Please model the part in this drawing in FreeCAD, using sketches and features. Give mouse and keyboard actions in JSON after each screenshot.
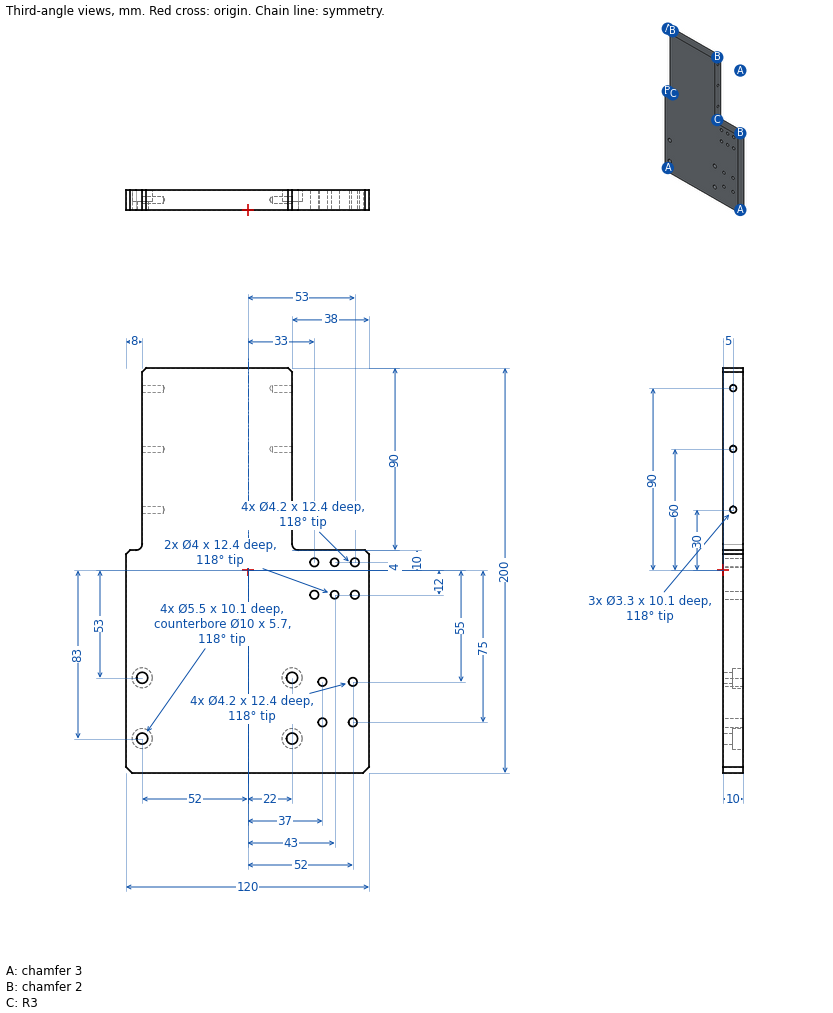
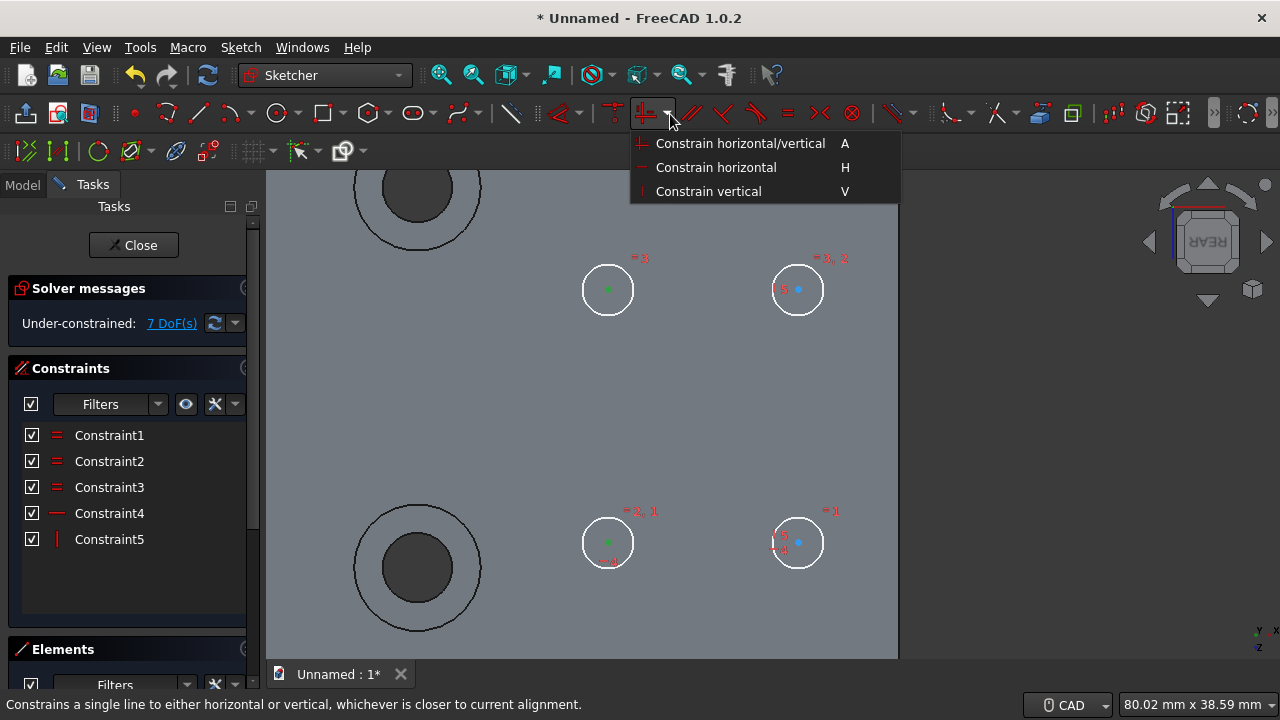
{"action": "left_click", "coordinate": [766, 191]}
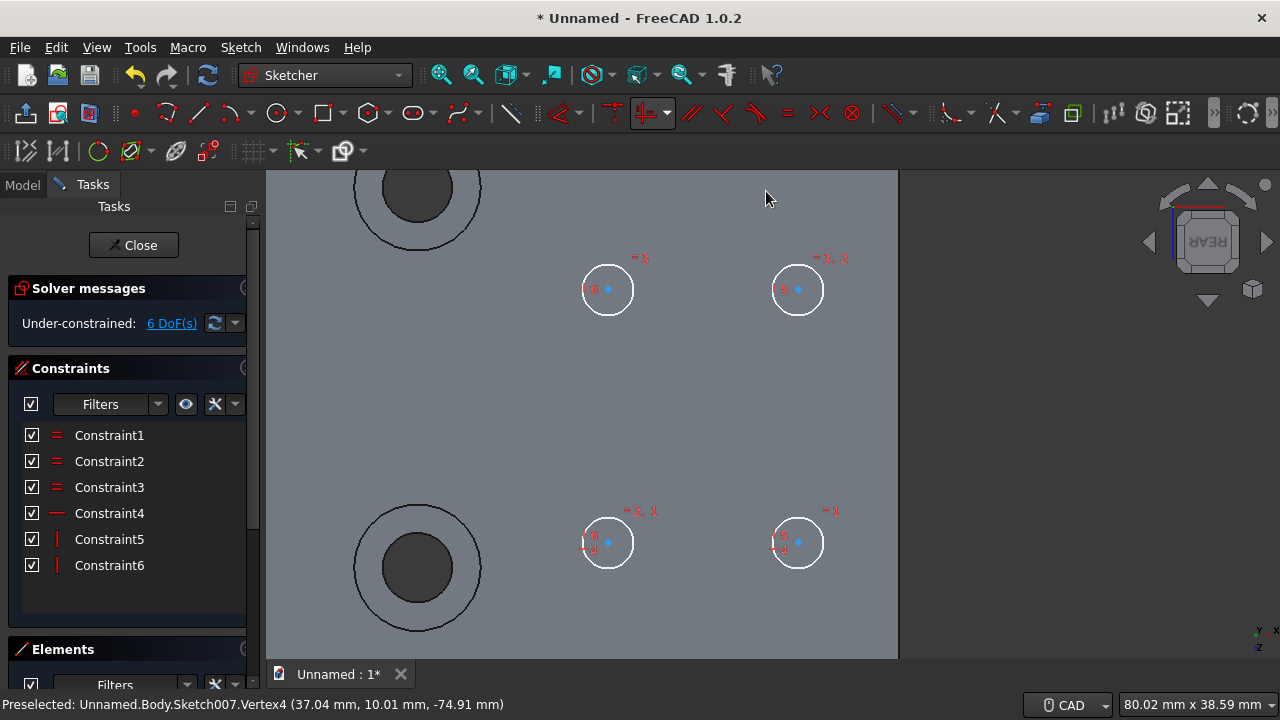
{"action": "left_click", "coordinate": [798, 290]}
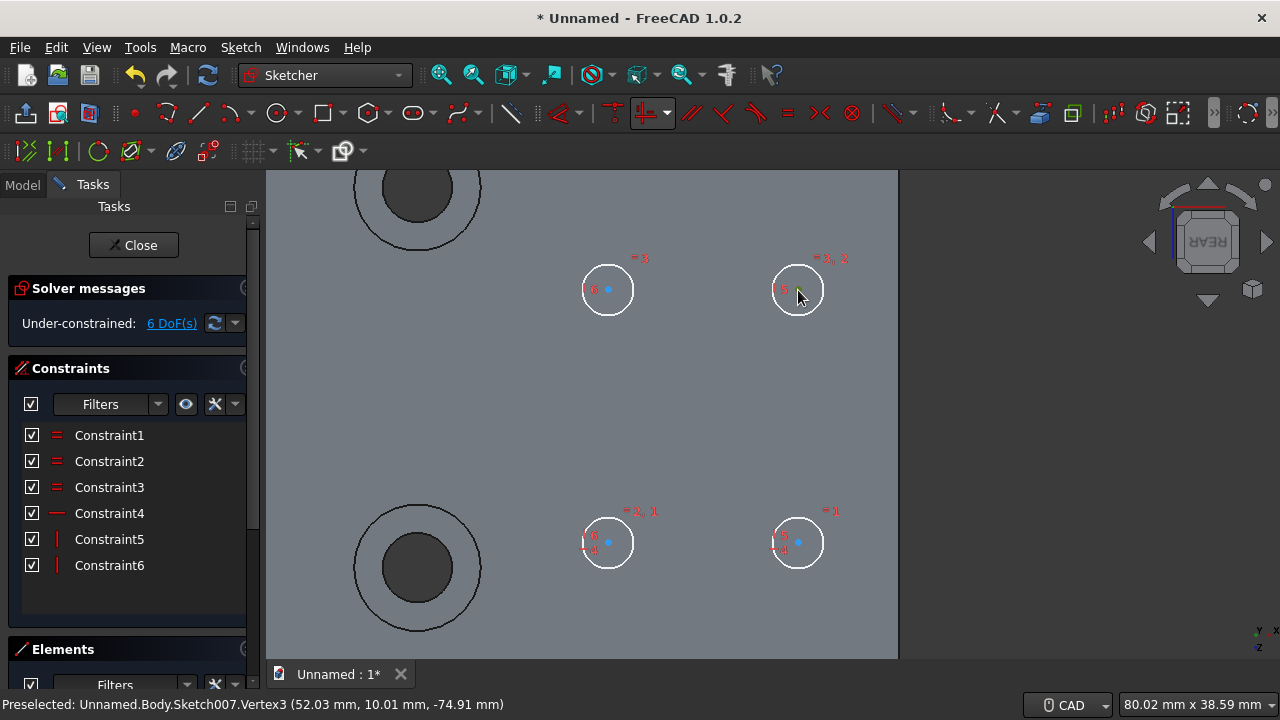
{"action": "left_click", "coordinate": [608, 290]}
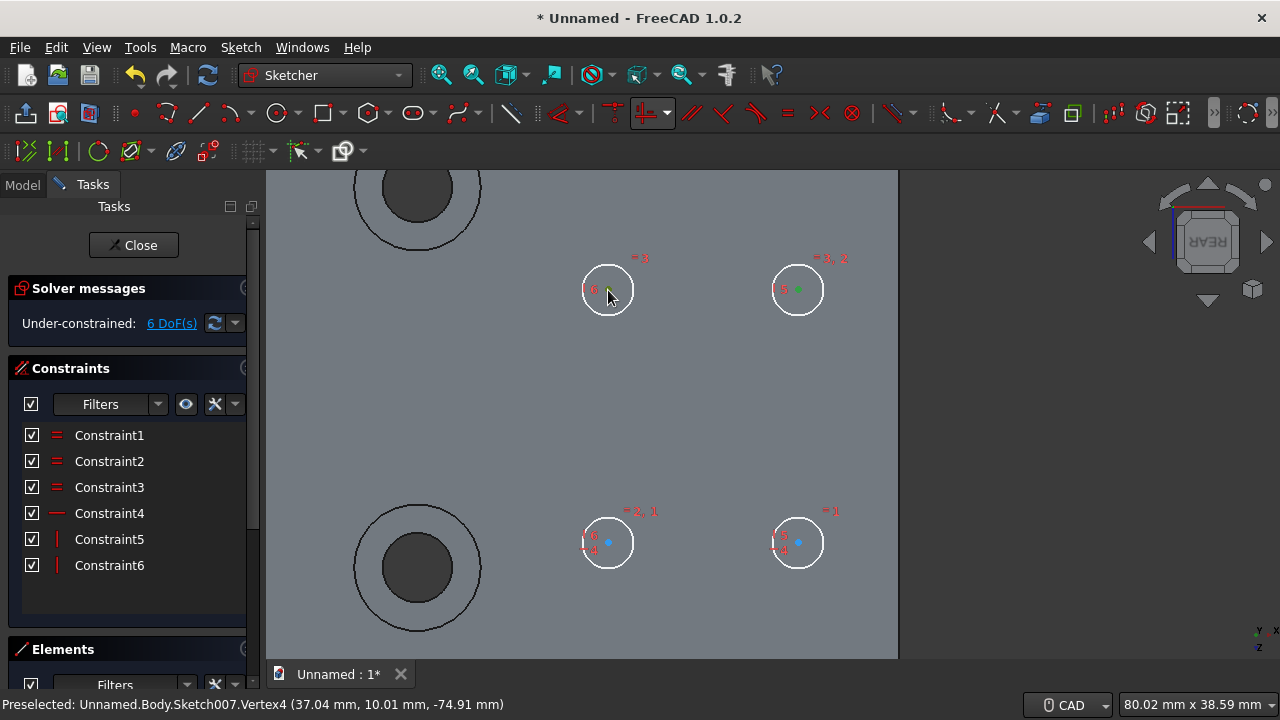
{"action": "key", "text": "h"}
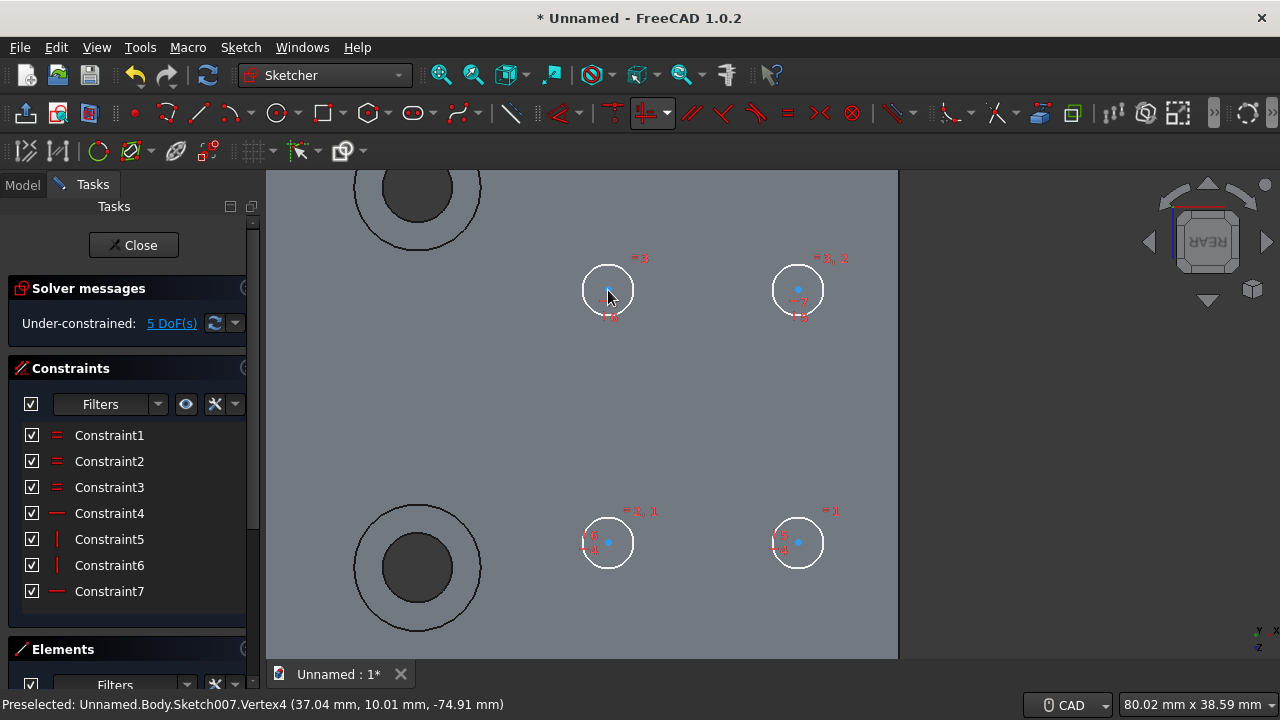
{"action": "key", "text": "d"}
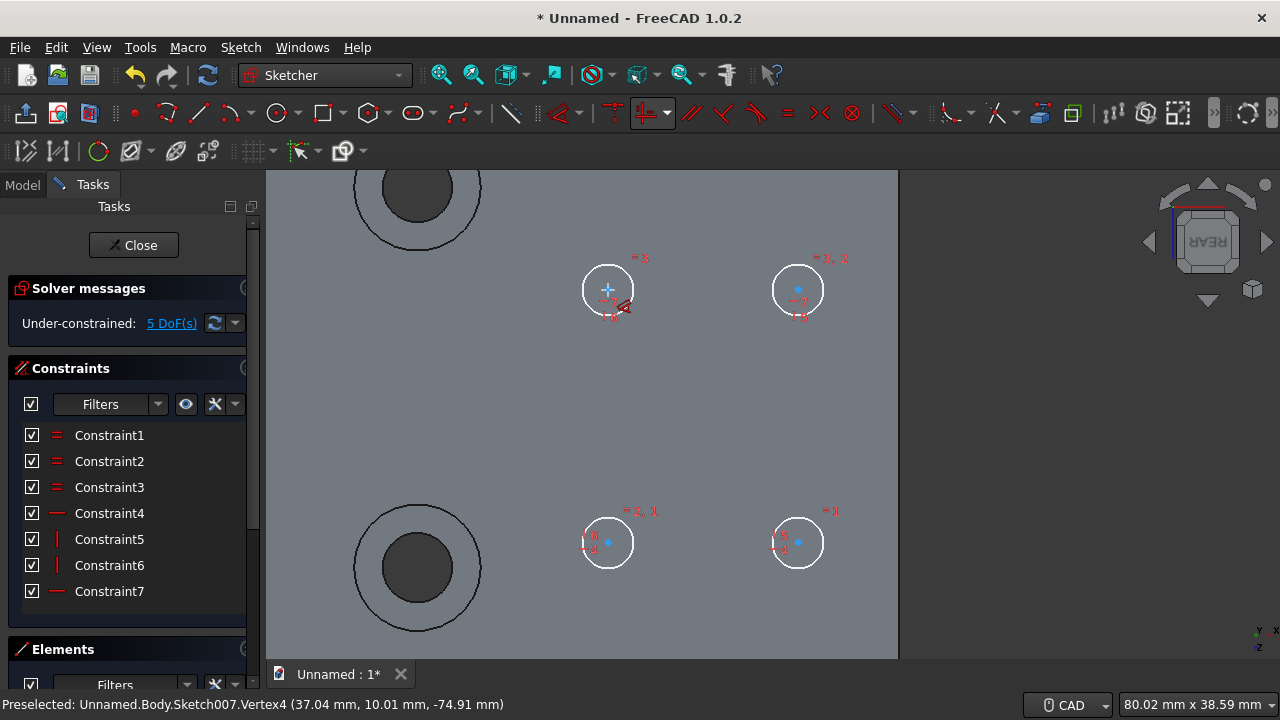
{"action": "left_click", "coordinate": [816, 525]}
{"action": "left_click", "coordinate": [839, 502]}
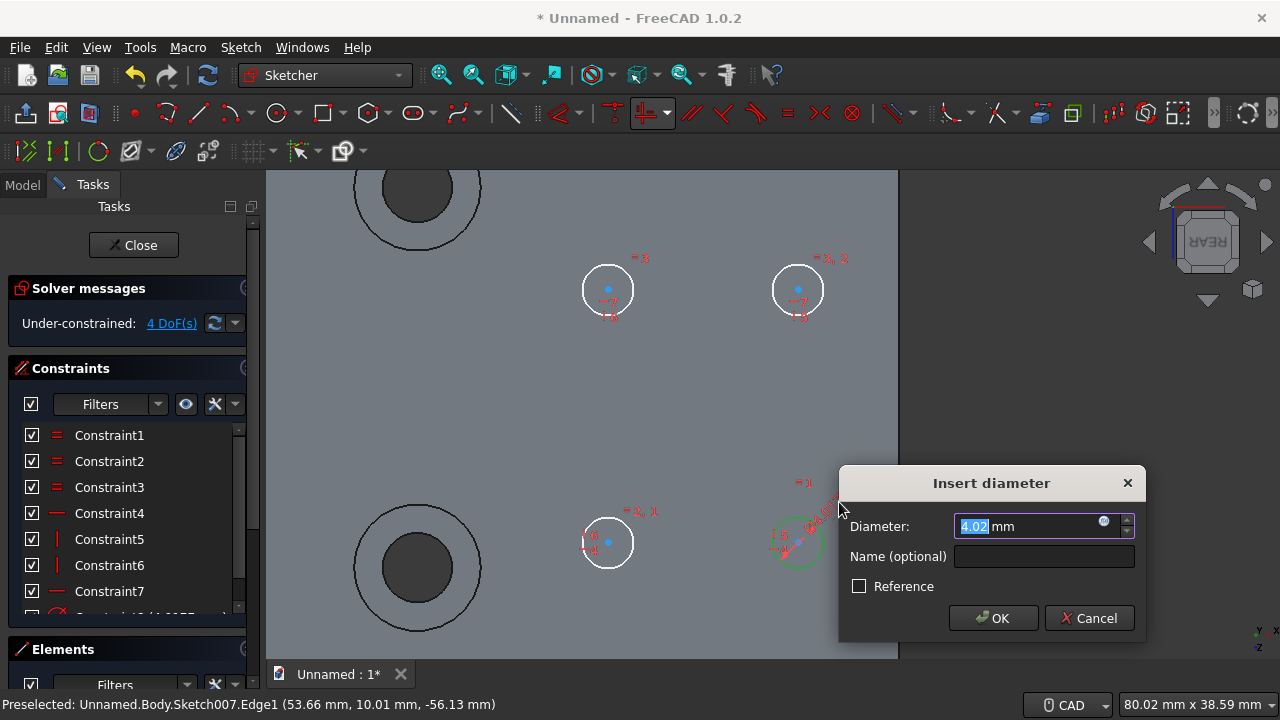
{"action": "type", "text": "4.2"}
{"action": "key", "text": "Return"}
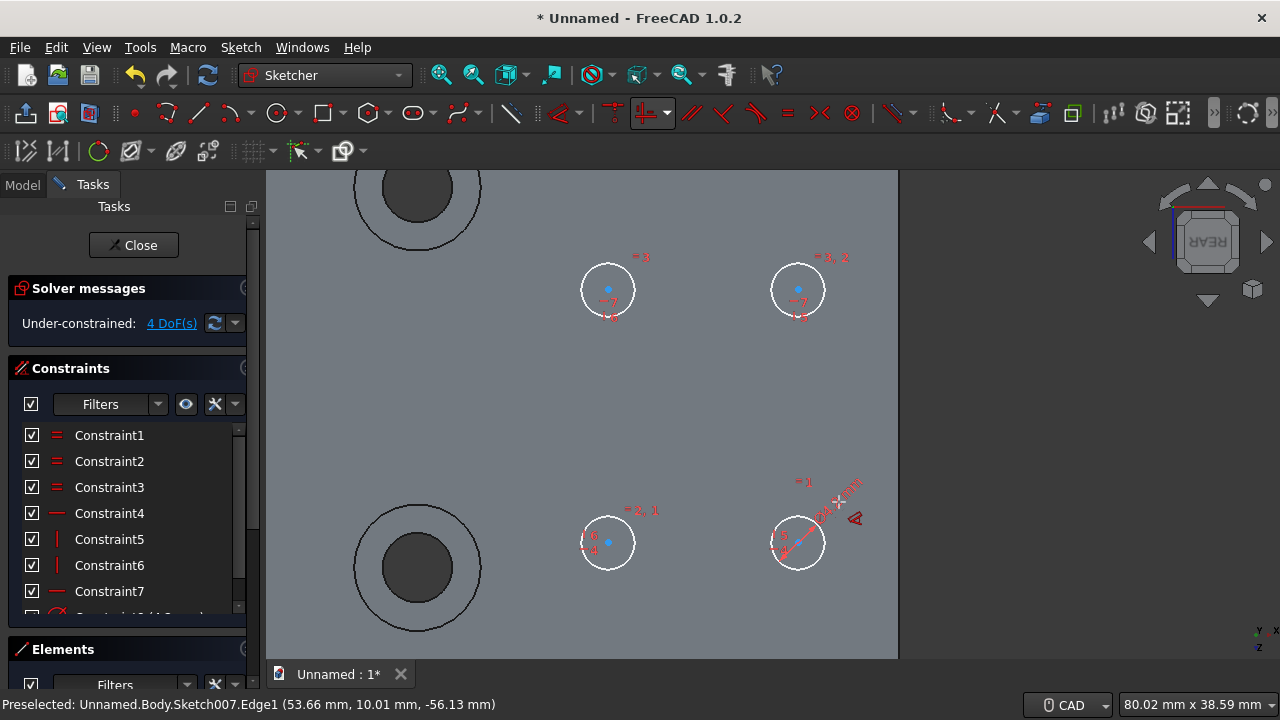
{"action": "left_click", "coordinate": [798, 543]}
{"action": "left_click", "coordinate": [546, 509]}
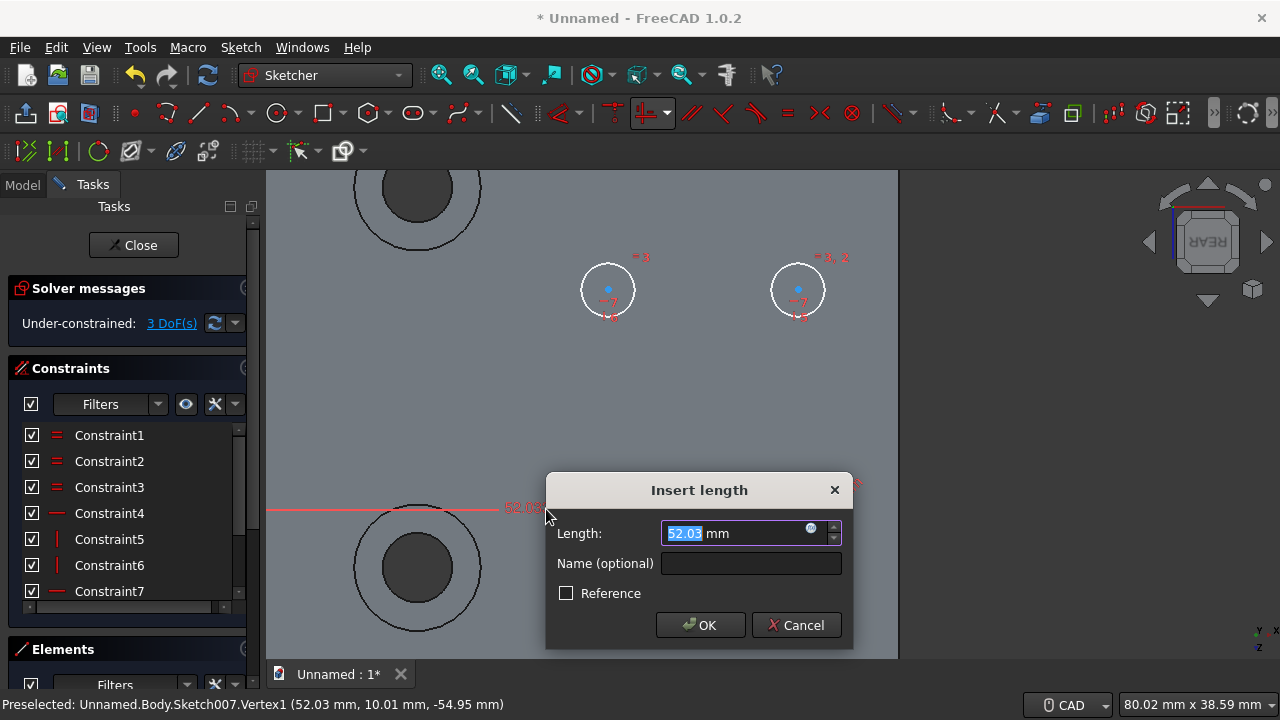
{"action": "type", "text": "52"}
{"action": "key", "text": "Return"}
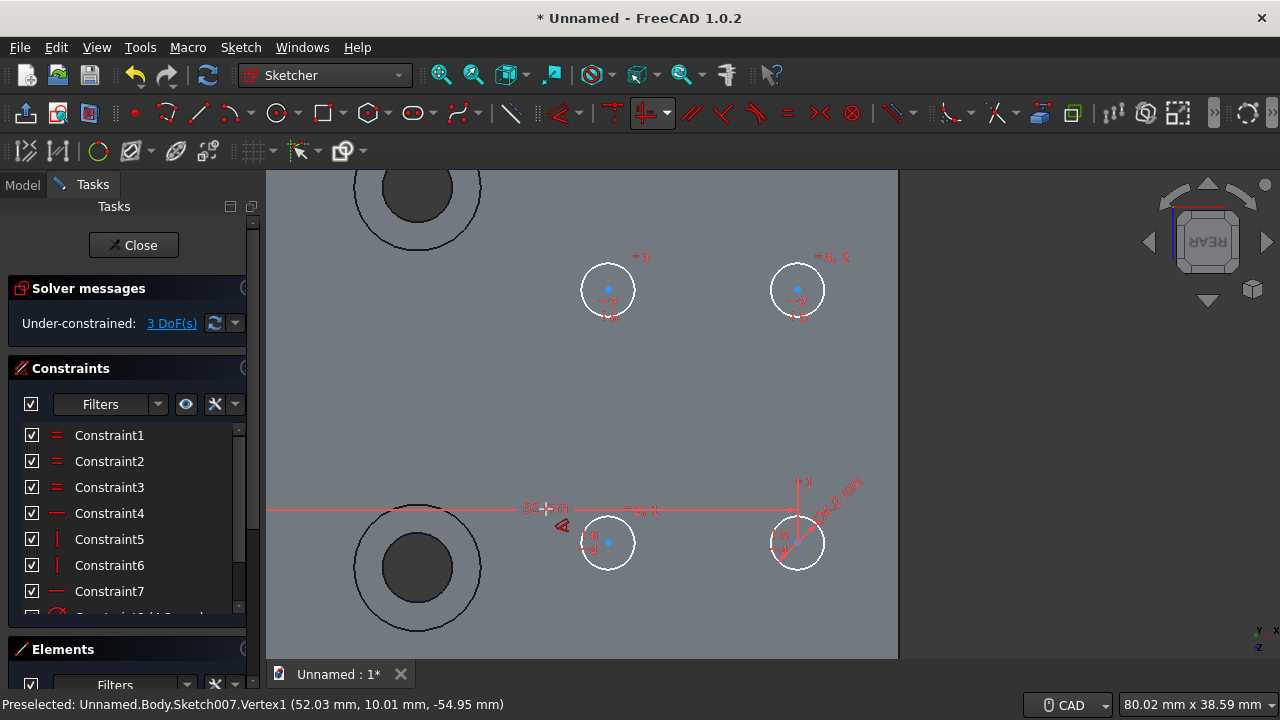
{"action": "left_click", "coordinate": [798, 543]}
{"action": "left_click", "coordinate": [832, 587]}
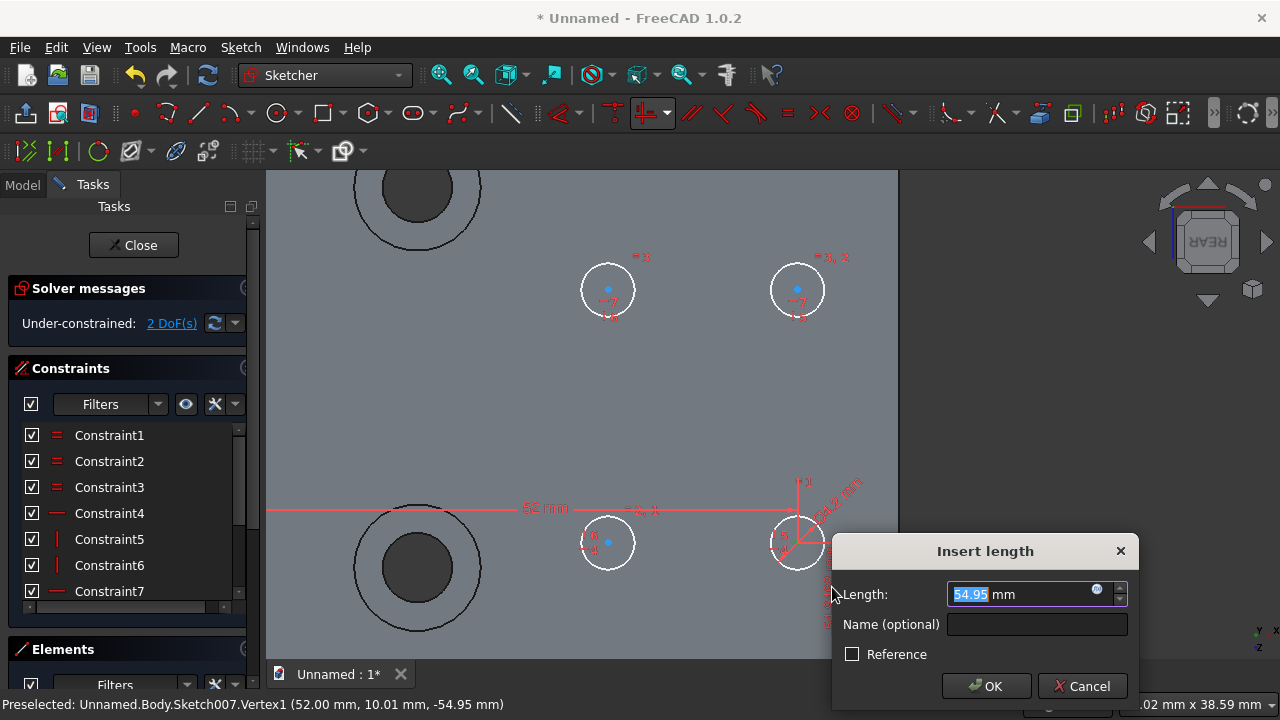
{"action": "type", "text": "55"}
{"action": "key", "text": "Return"}